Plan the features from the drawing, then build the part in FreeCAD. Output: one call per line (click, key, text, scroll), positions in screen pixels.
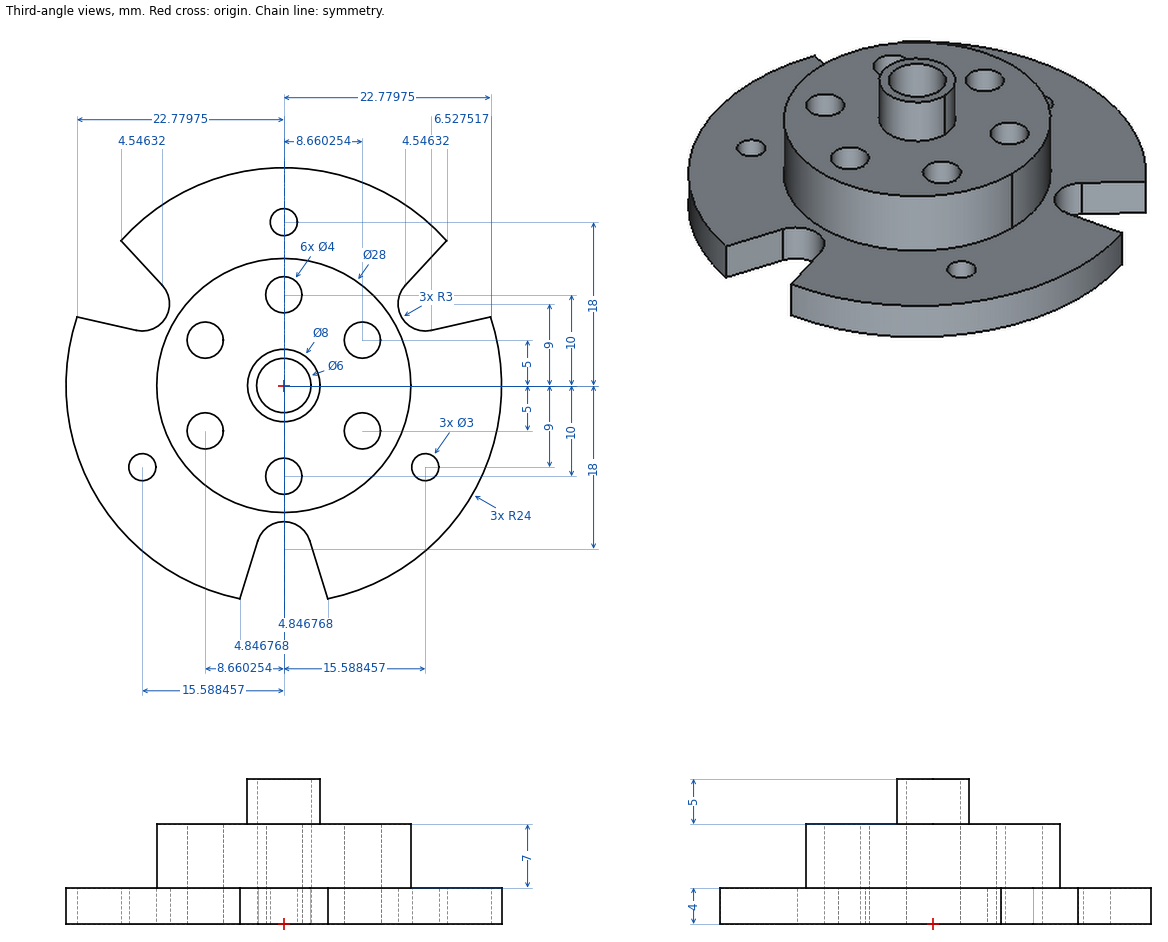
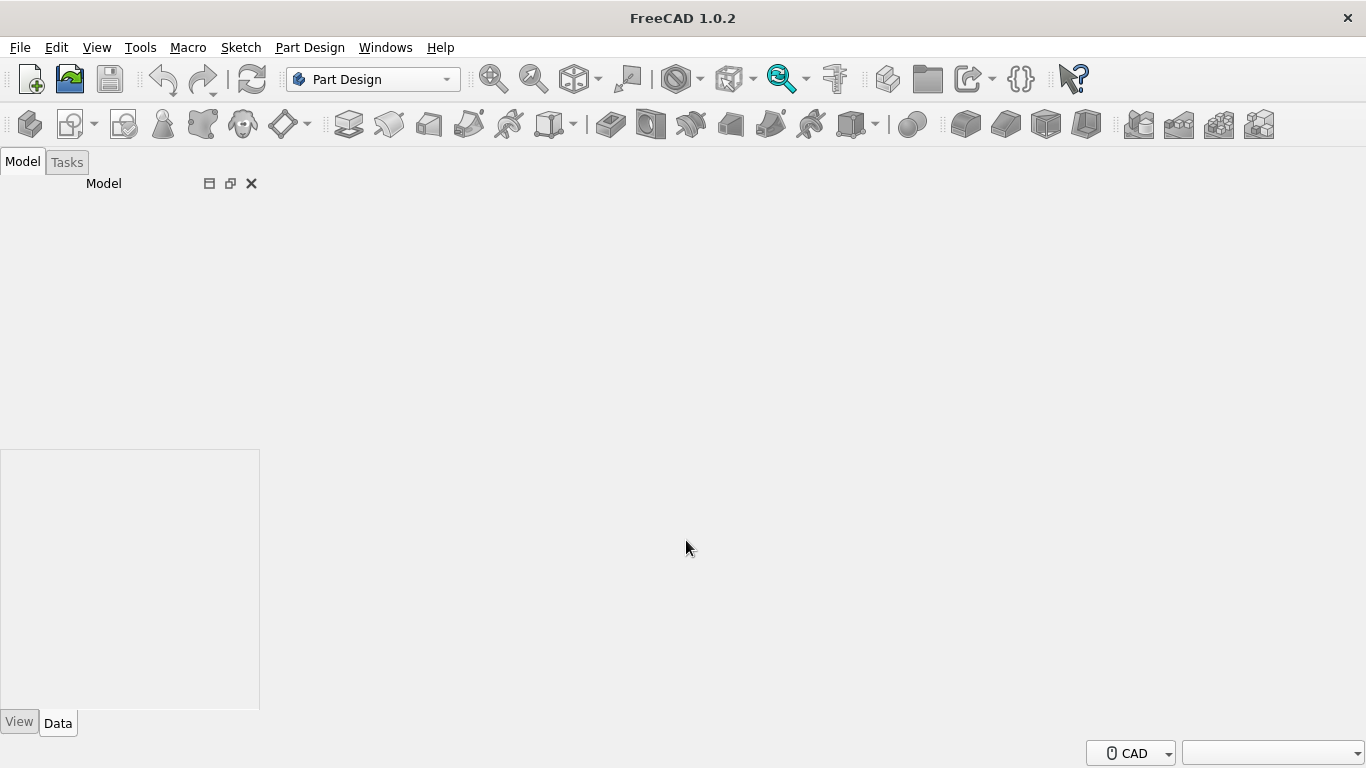
click(30, 80)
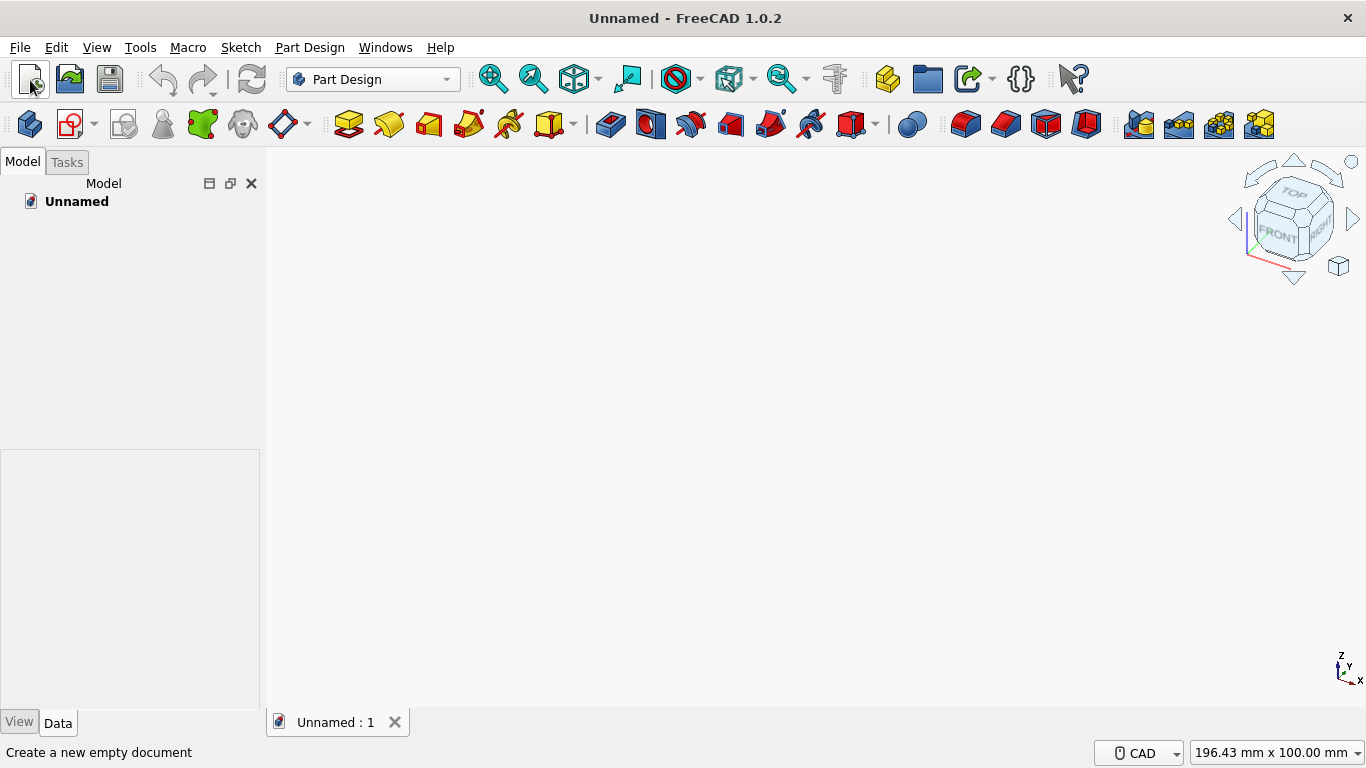
click(70, 124)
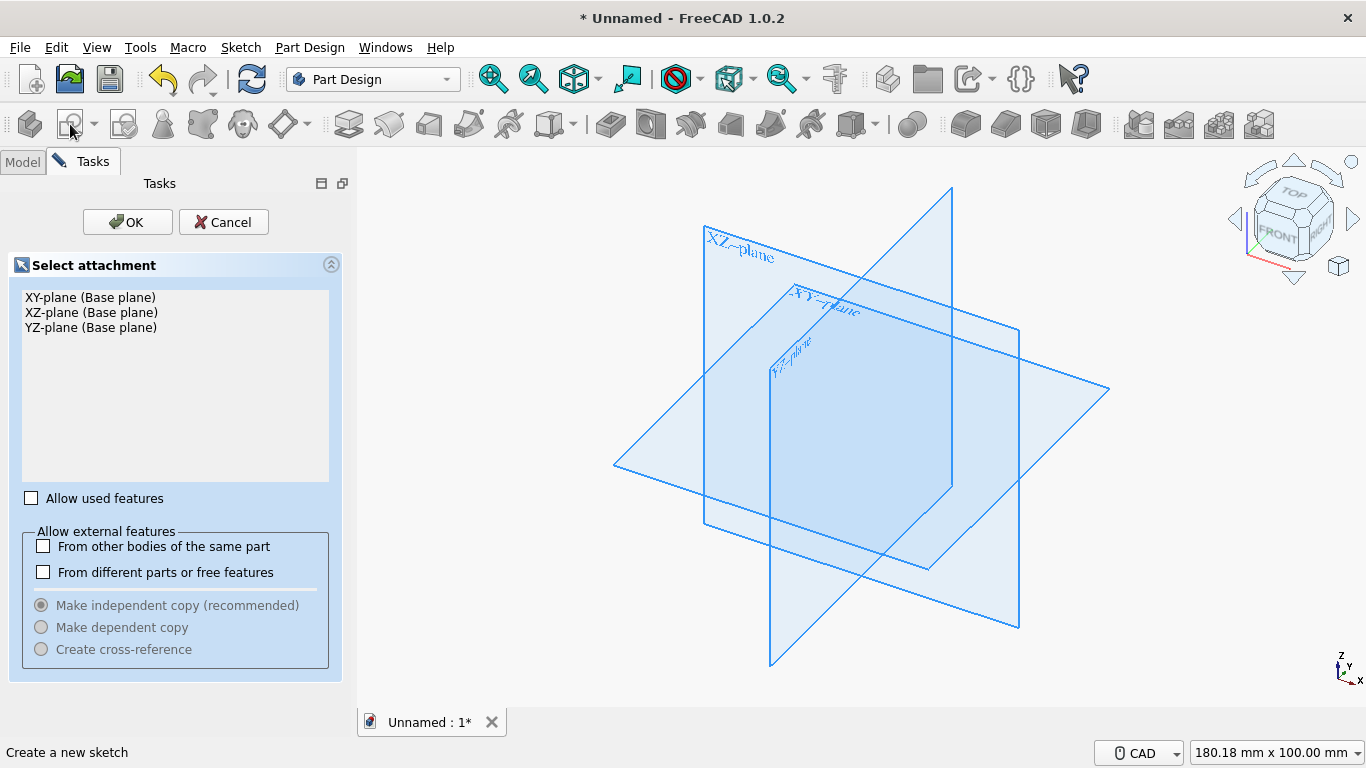
click(82, 298)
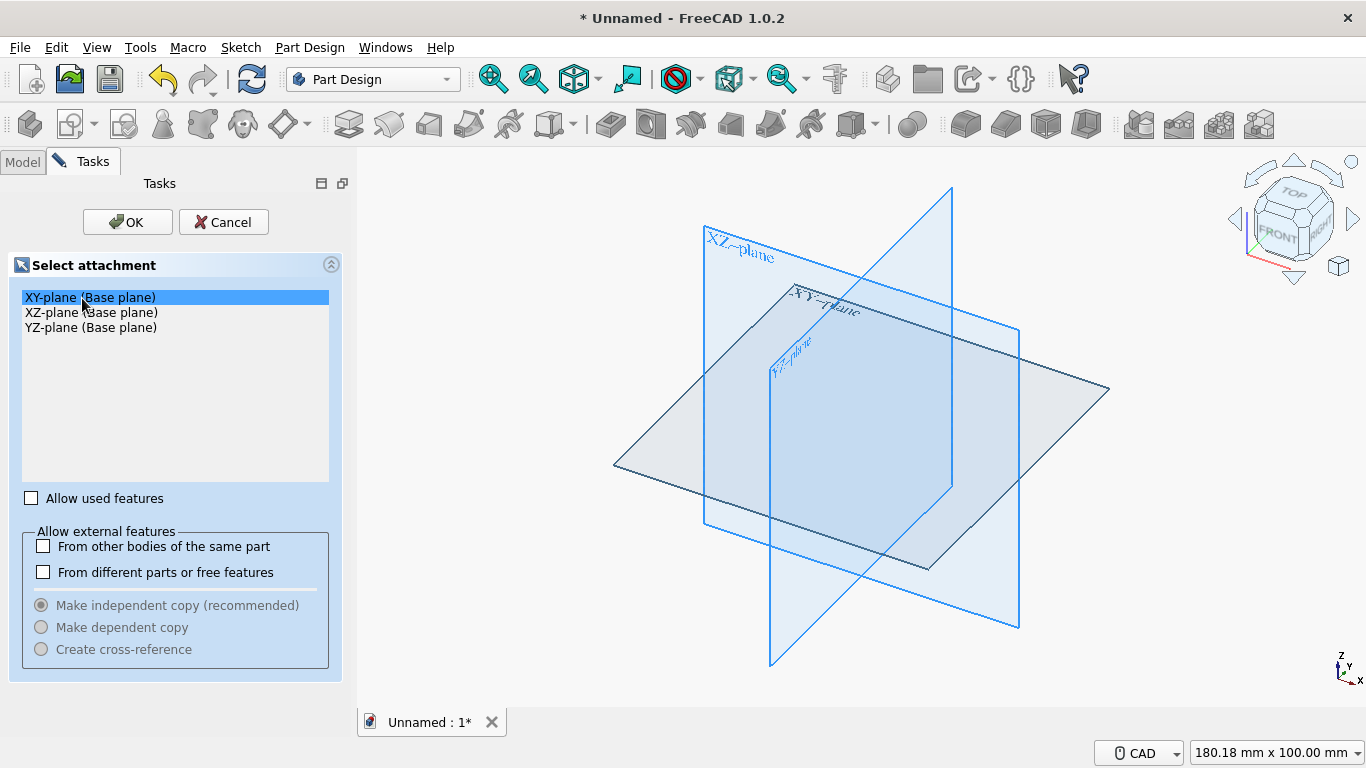
click(128, 222)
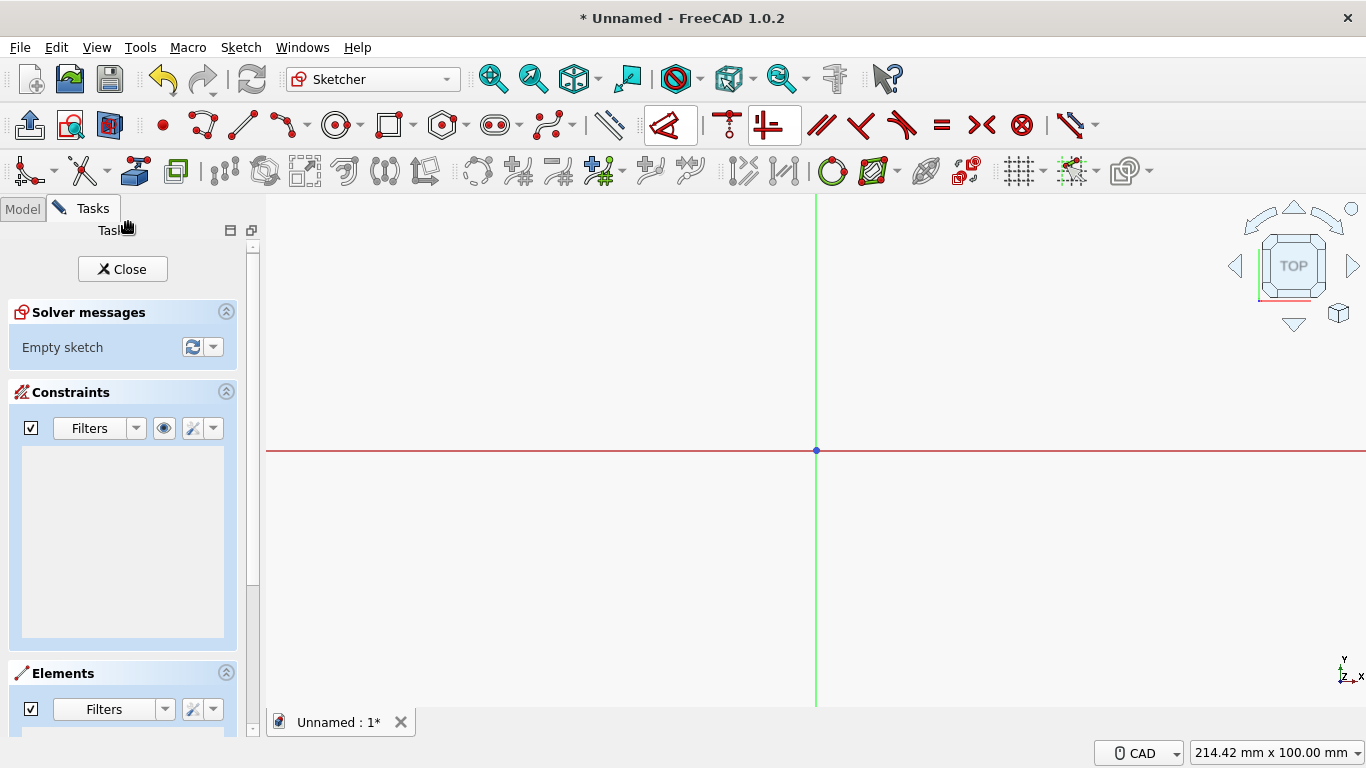
key(g)
key(l)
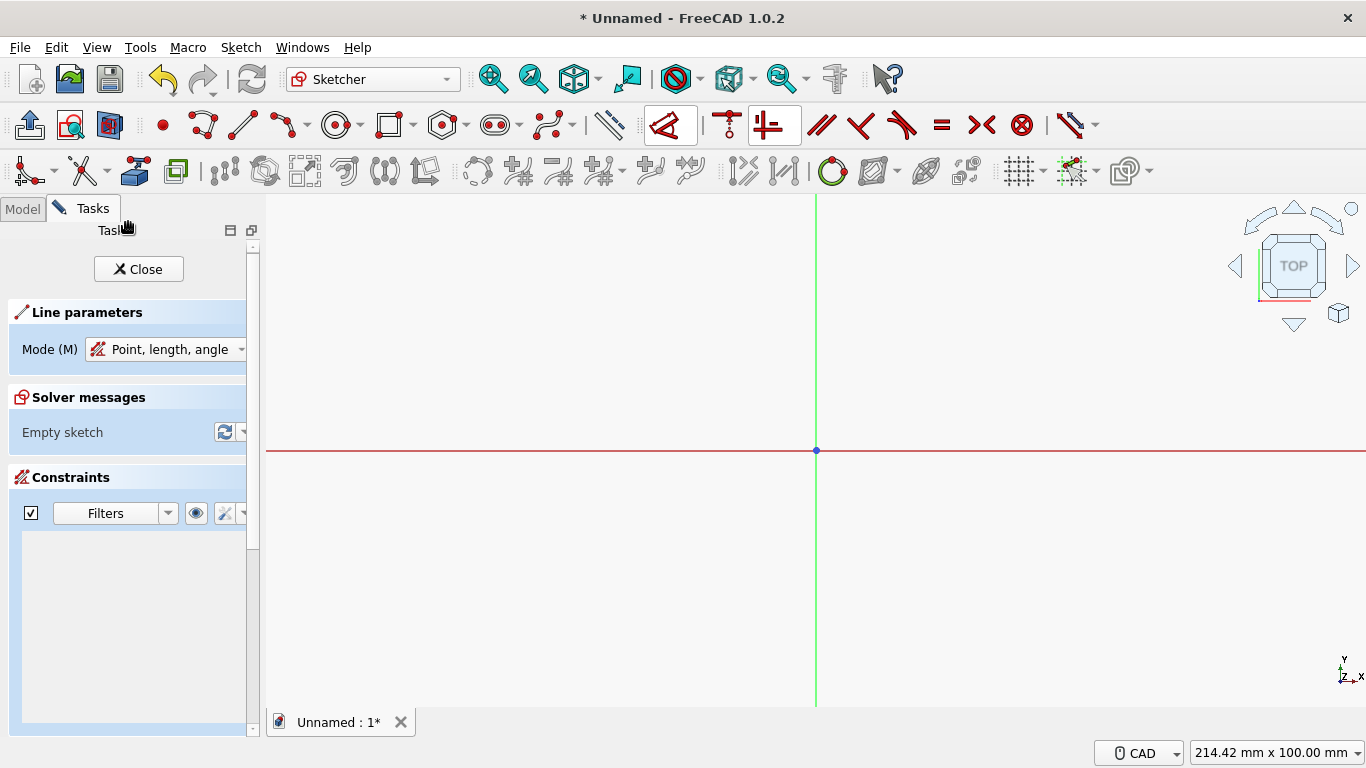
click(831, 538)
click(841, 571)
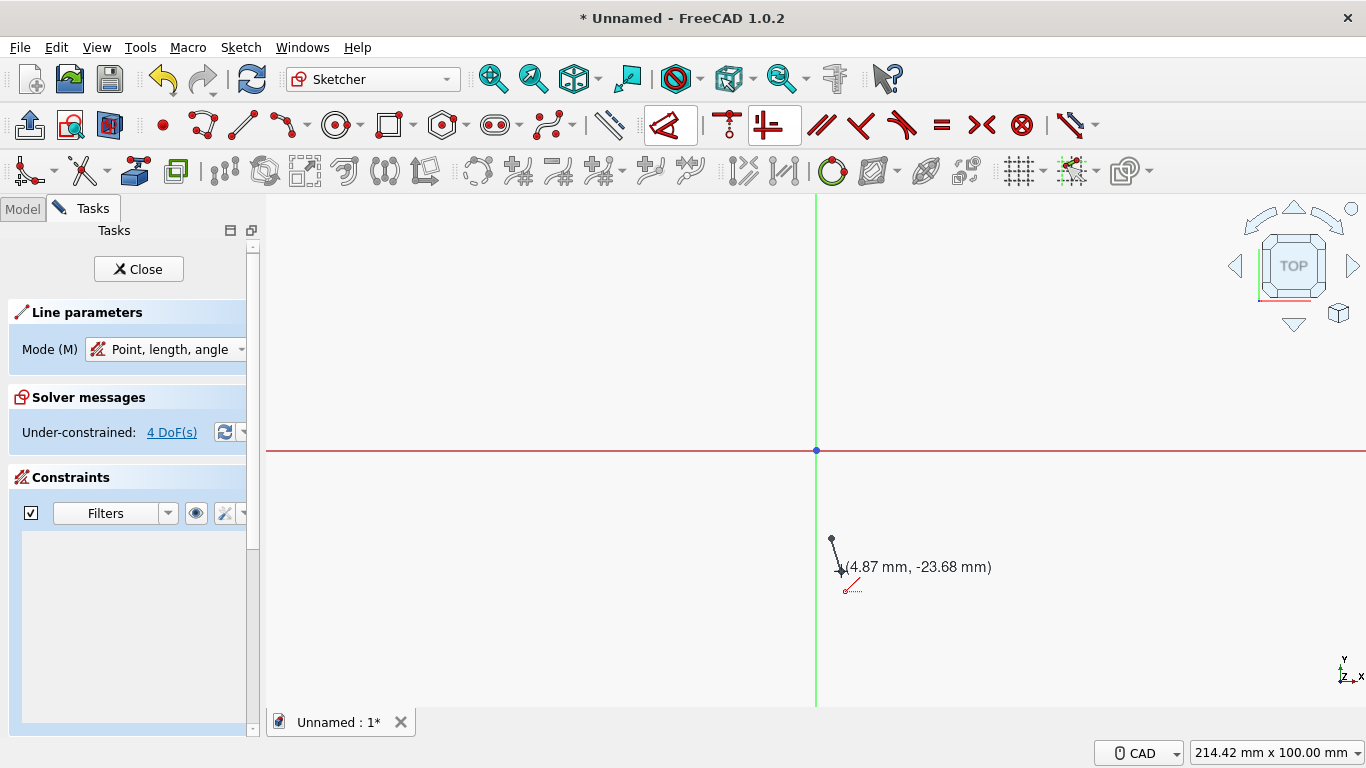
click(933, 412)
click(899, 419)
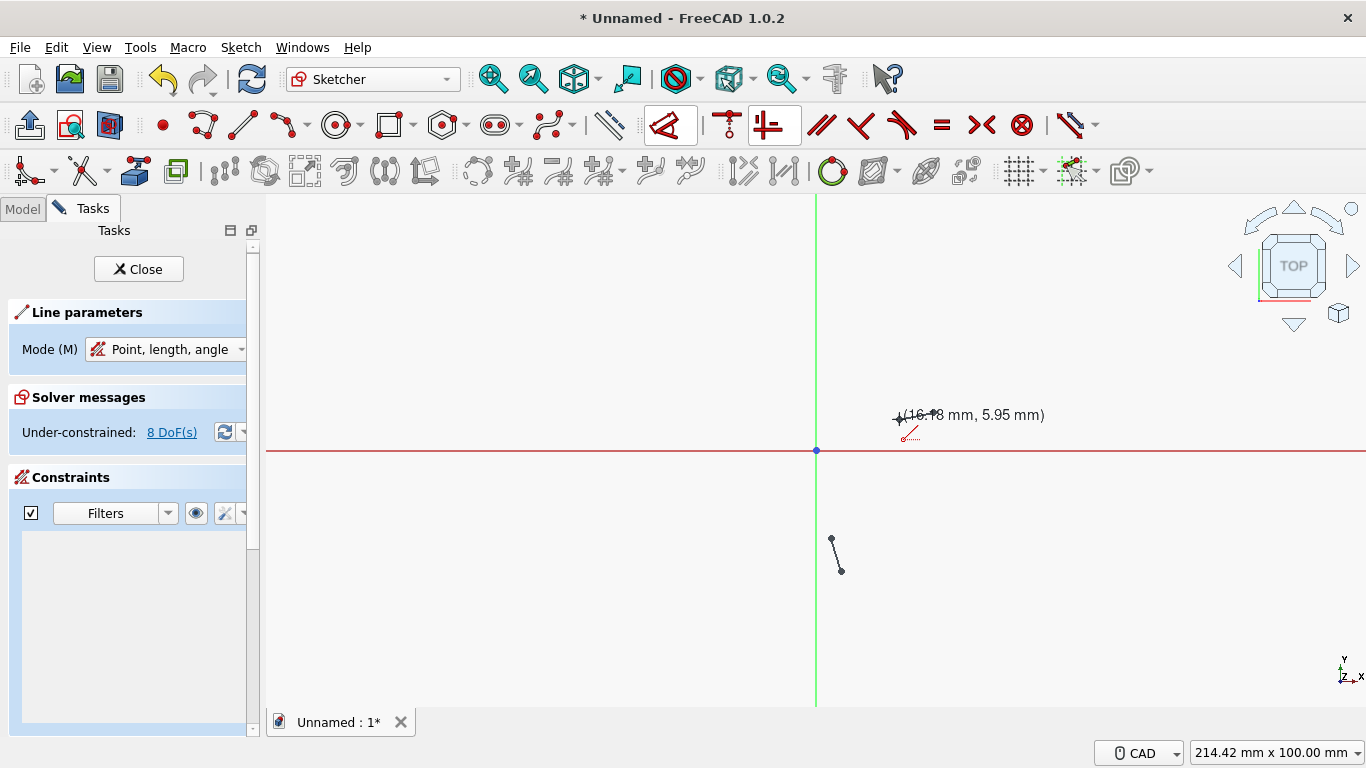
click(885, 394)
click(908, 369)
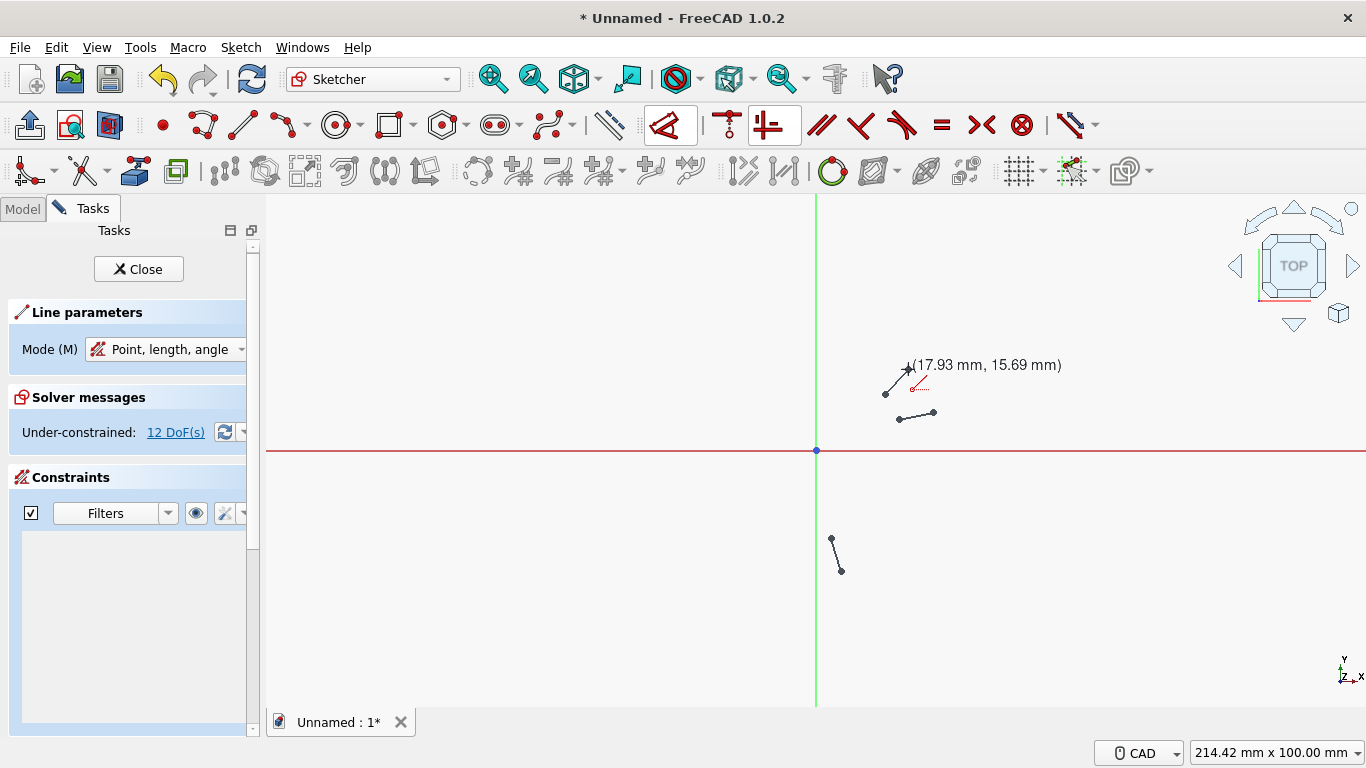
click(724, 369)
click(747, 394)